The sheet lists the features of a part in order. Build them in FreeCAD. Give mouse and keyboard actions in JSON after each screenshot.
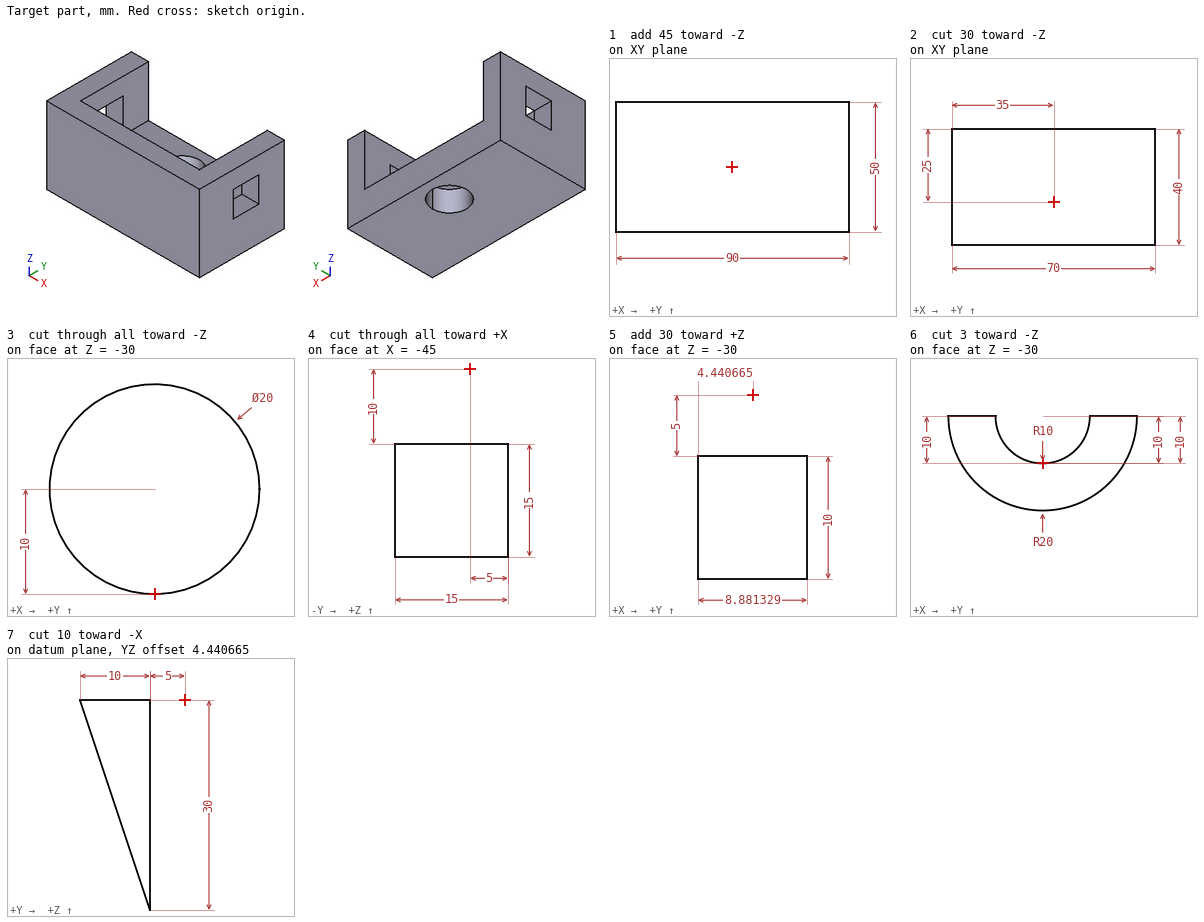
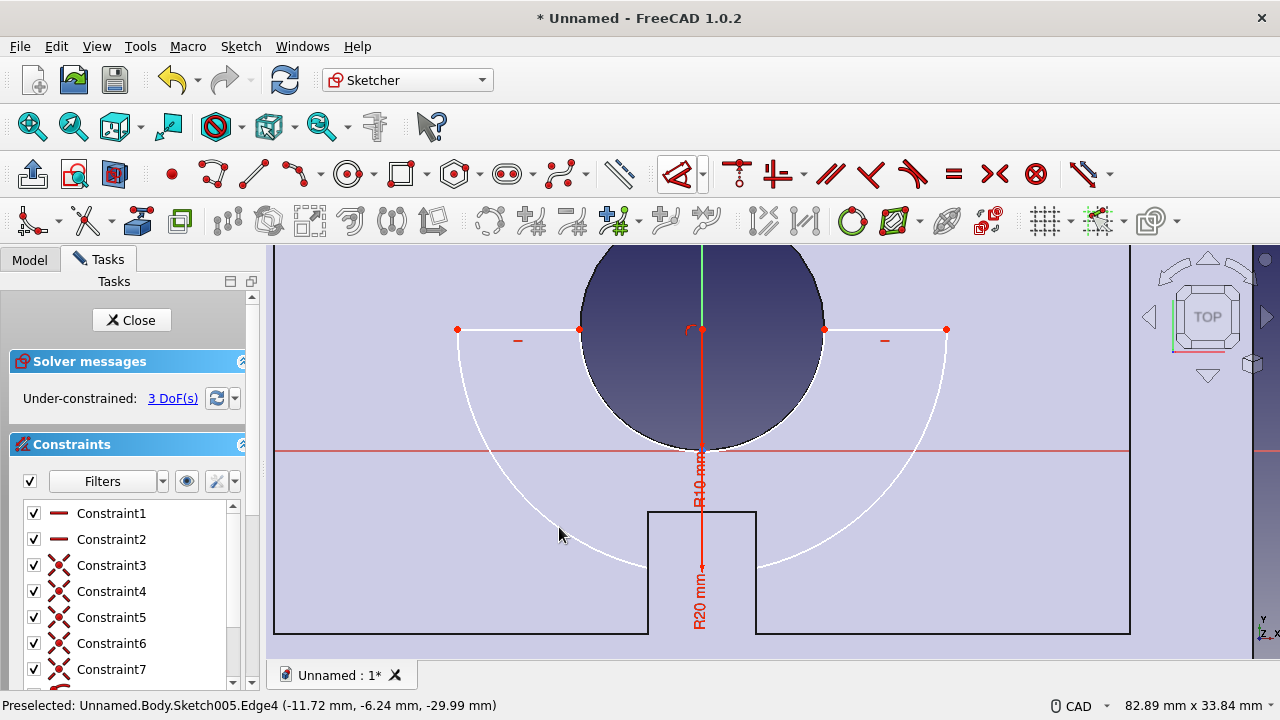
{"action": "left_click", "coordinate": [947, 330]}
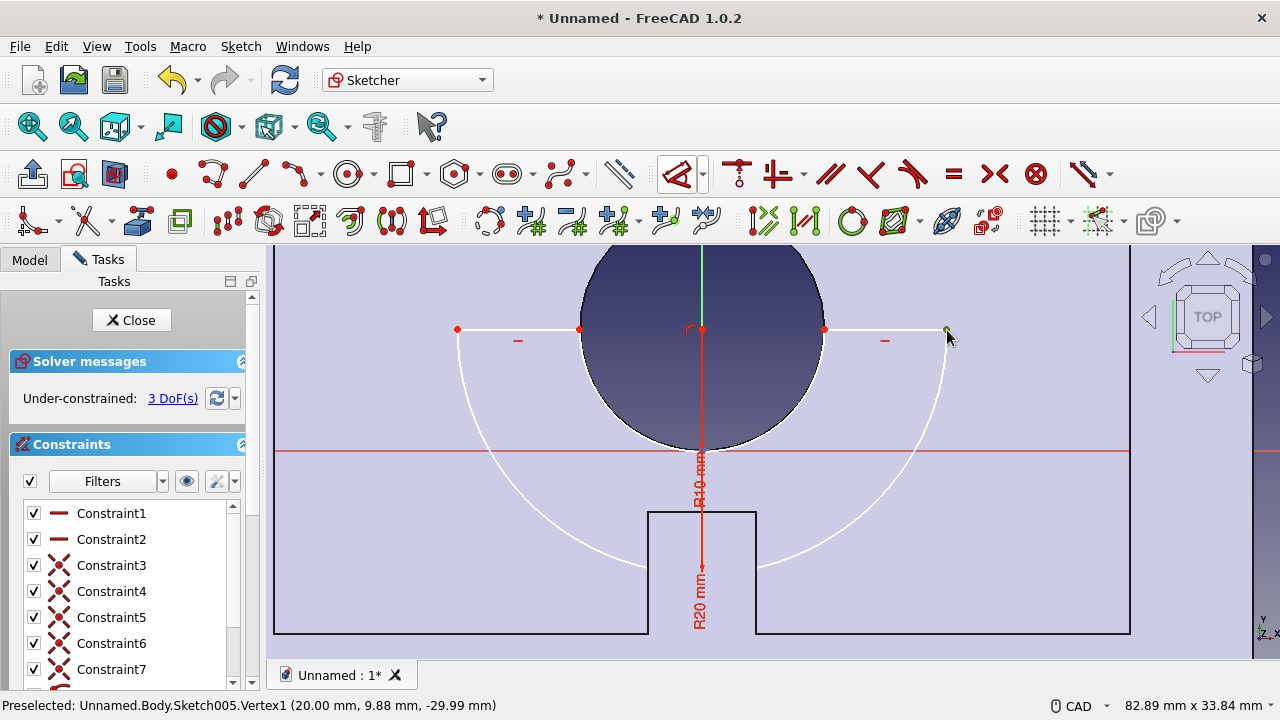
{"action": "key", "text": "i"}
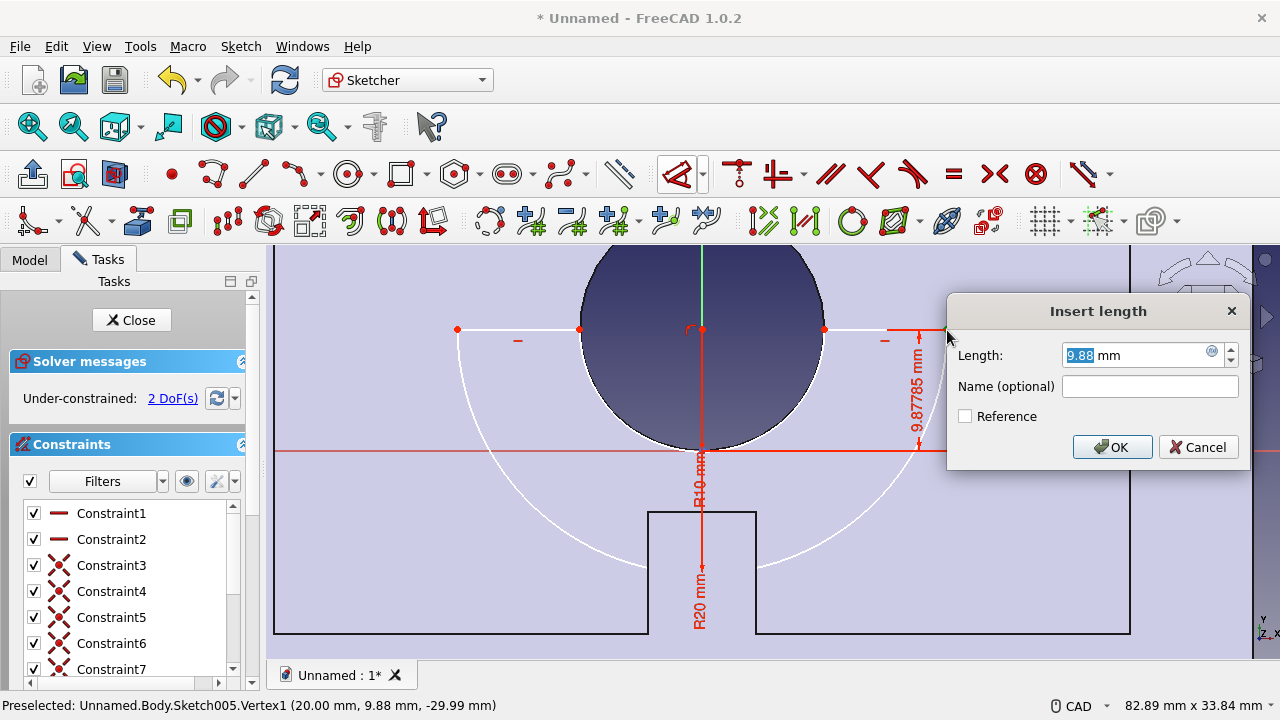
{"action": "type", "text": "10"}
{"action": "key", "text": "Return"}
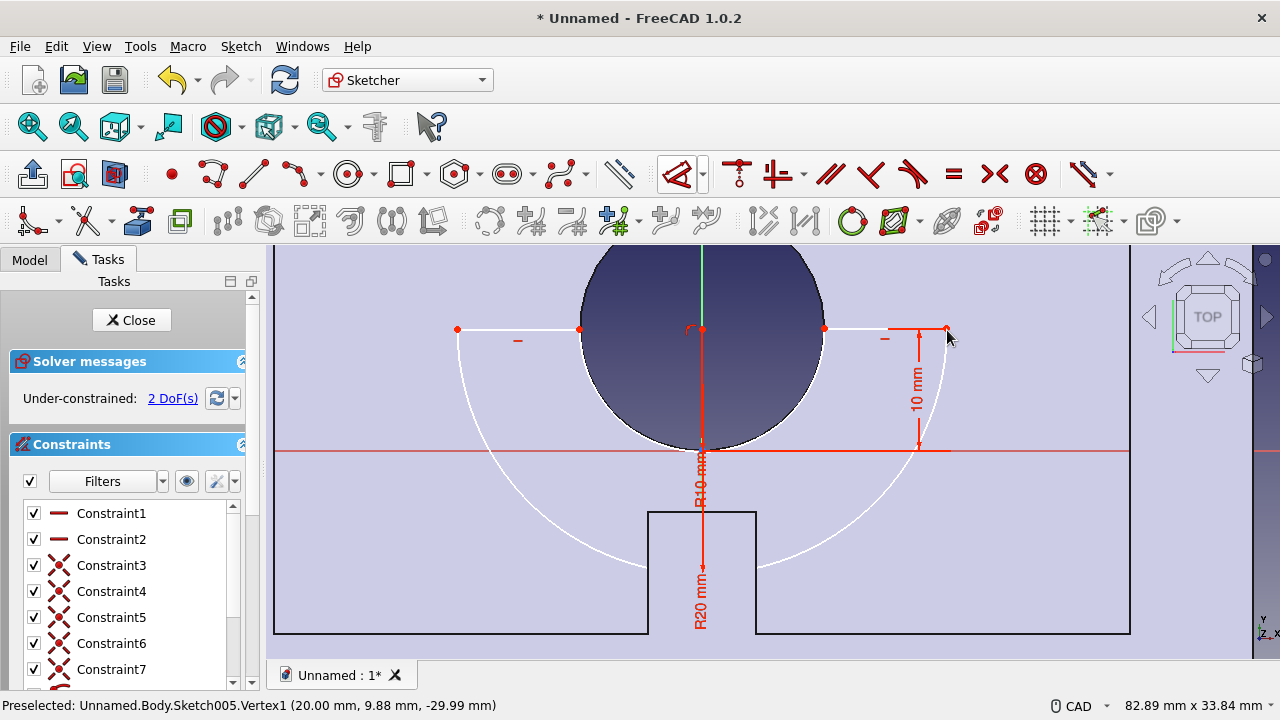
{"action": "left_click", "coordinate": [580, 330]}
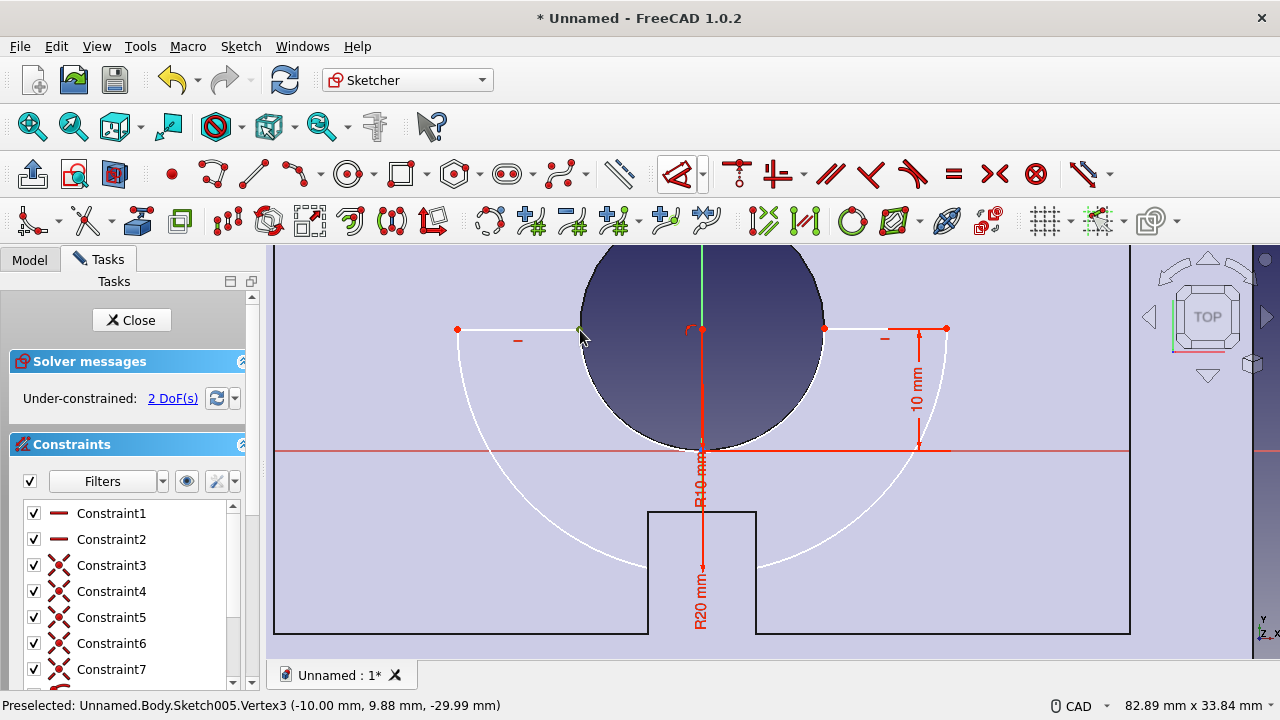
{"action": "key", "text": "i"}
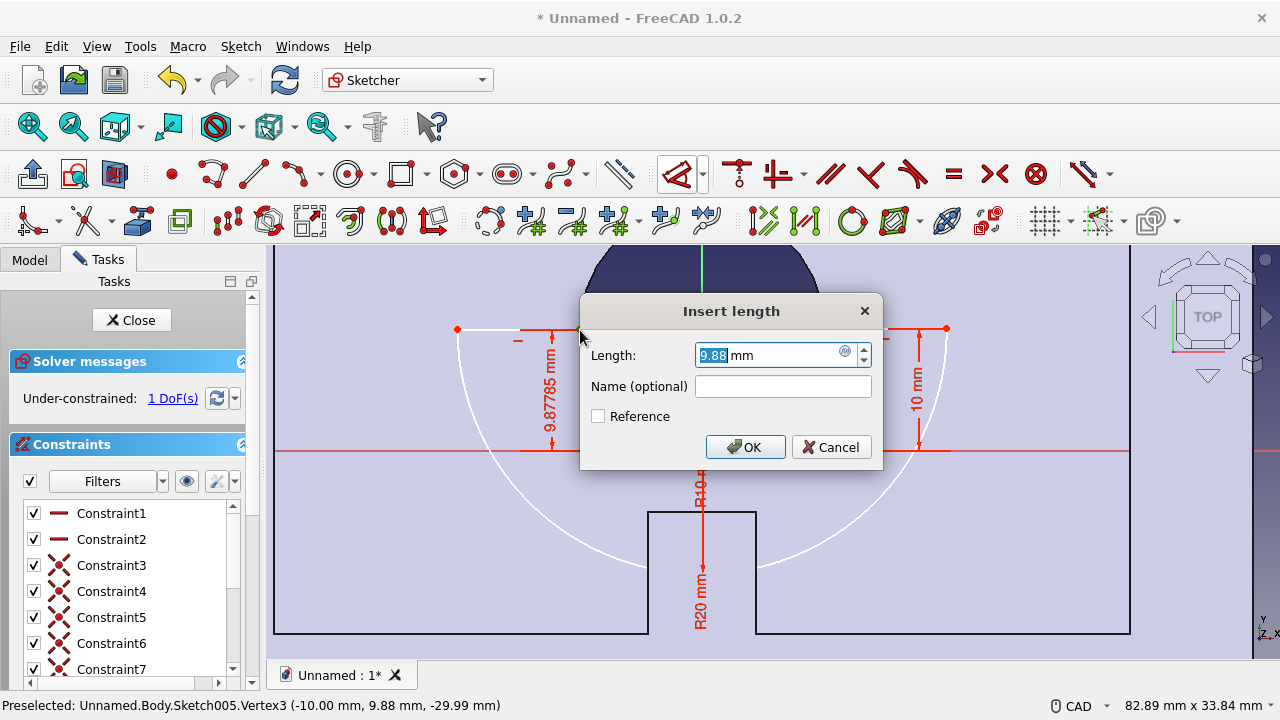
{"action": "type", "text": "10"}
{"action": "key", "text": "Return"}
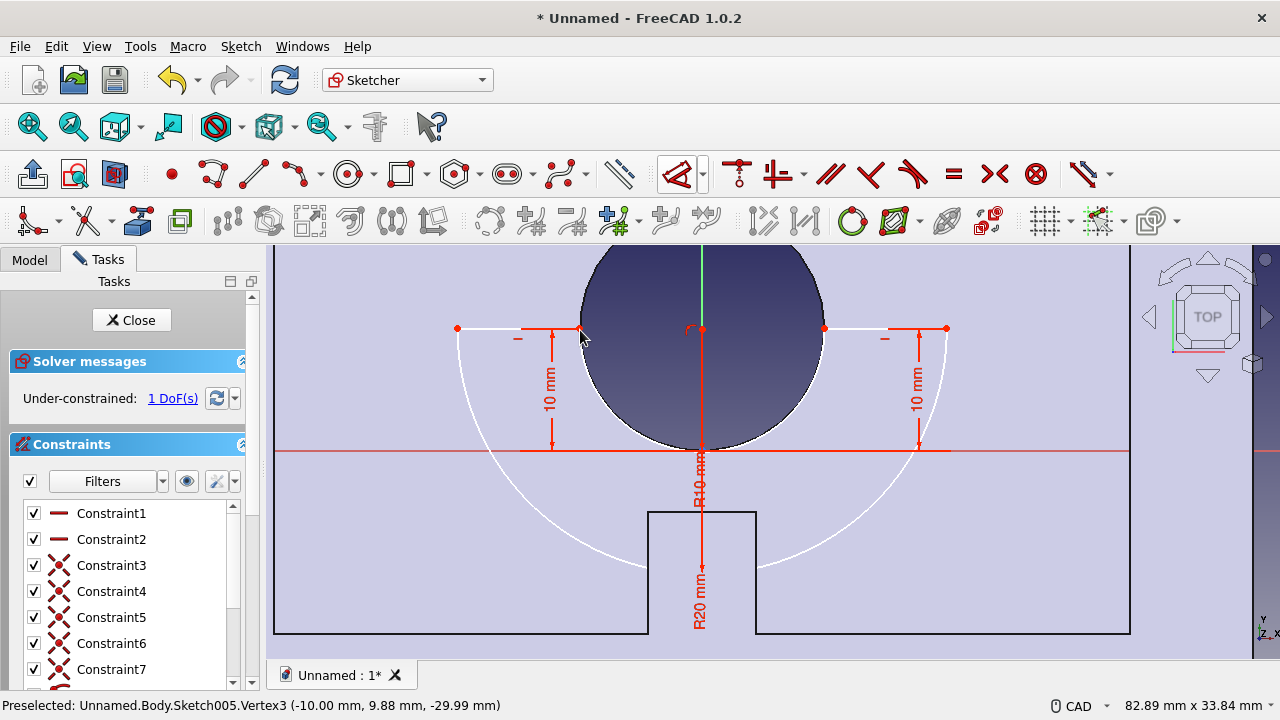
{"action": "left_click", "coordinate": [702, 329]}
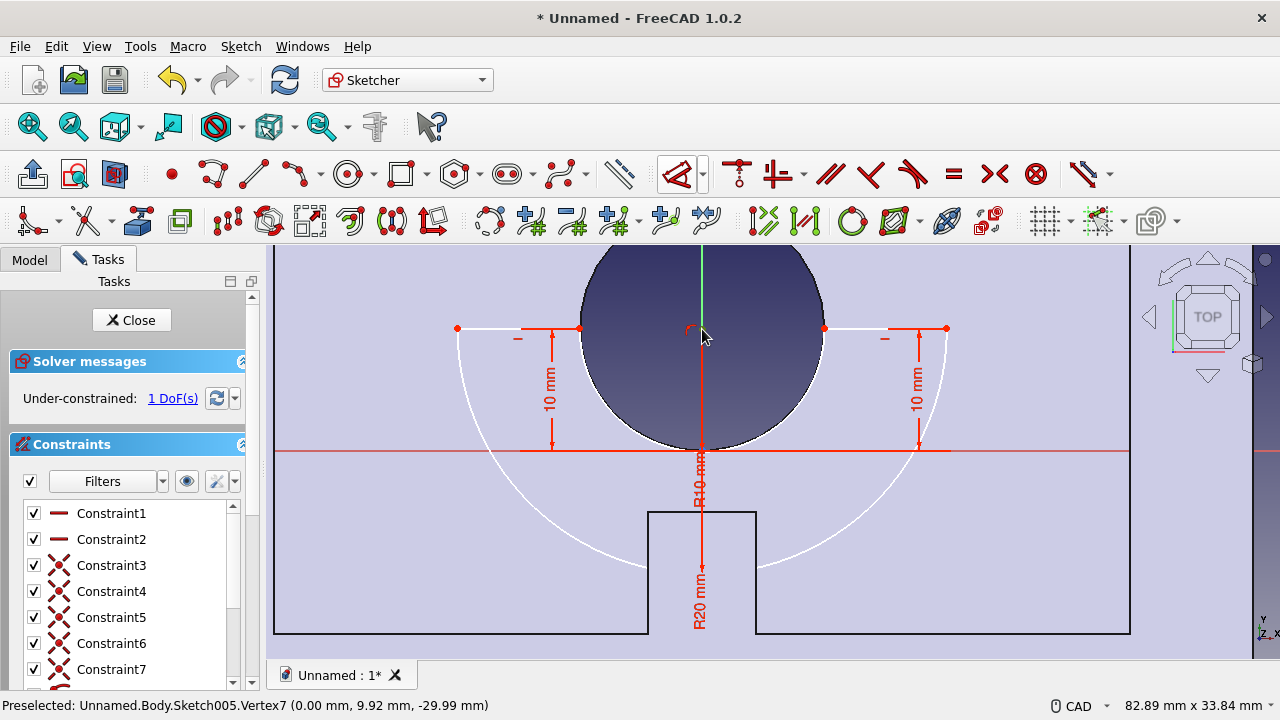
{"action": "key", "text": "i"}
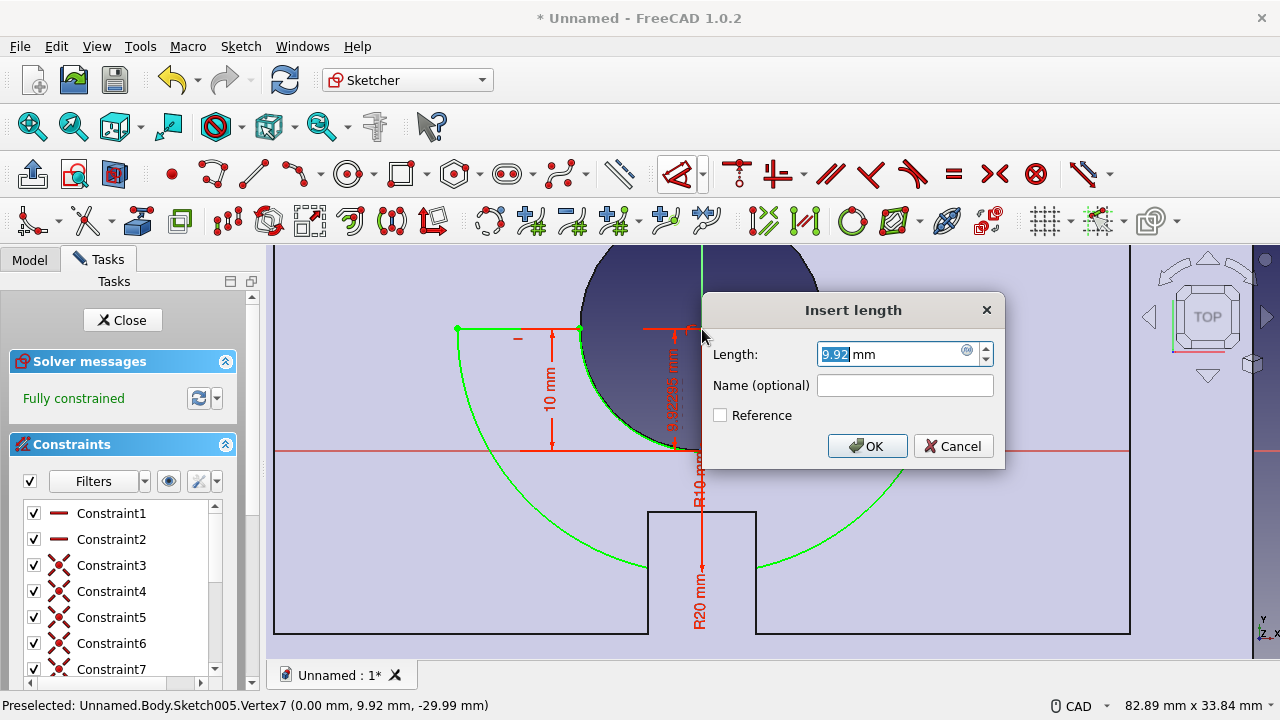
{"action": "type", "text": "10"}
{"action": "key", "text": "Return"}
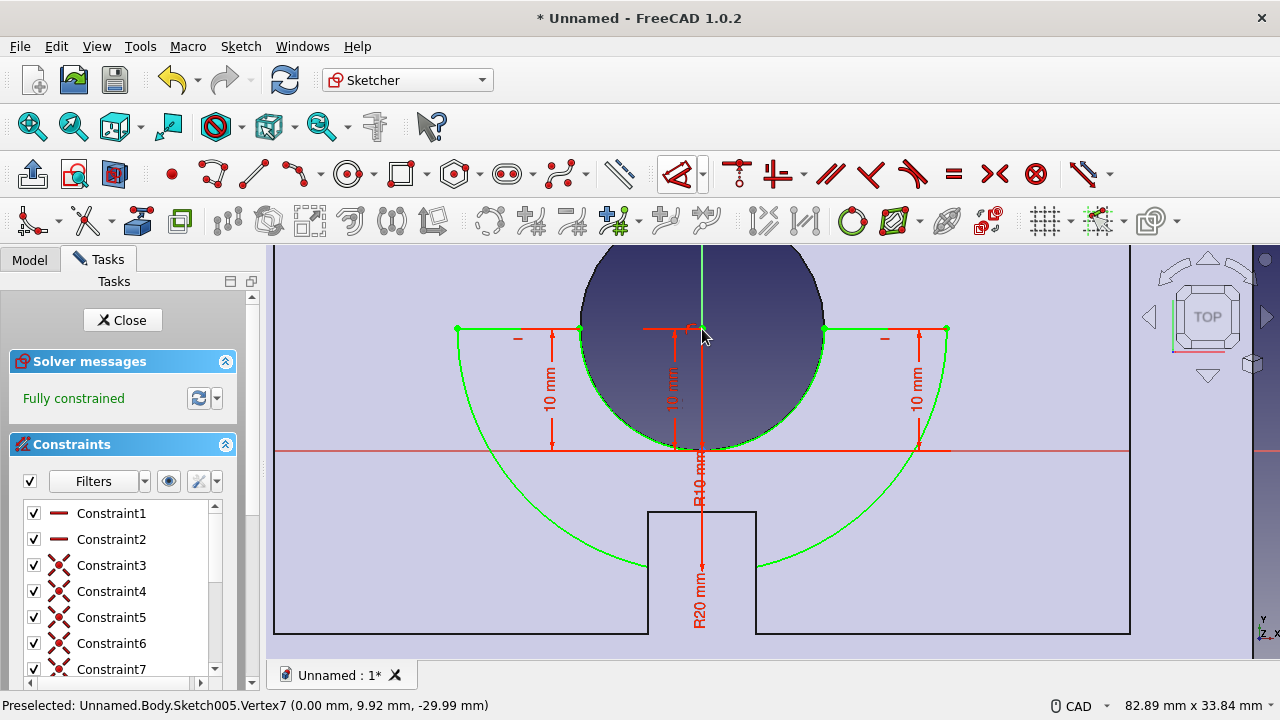
{"action": "left_click", "coordinate": [123, 320]}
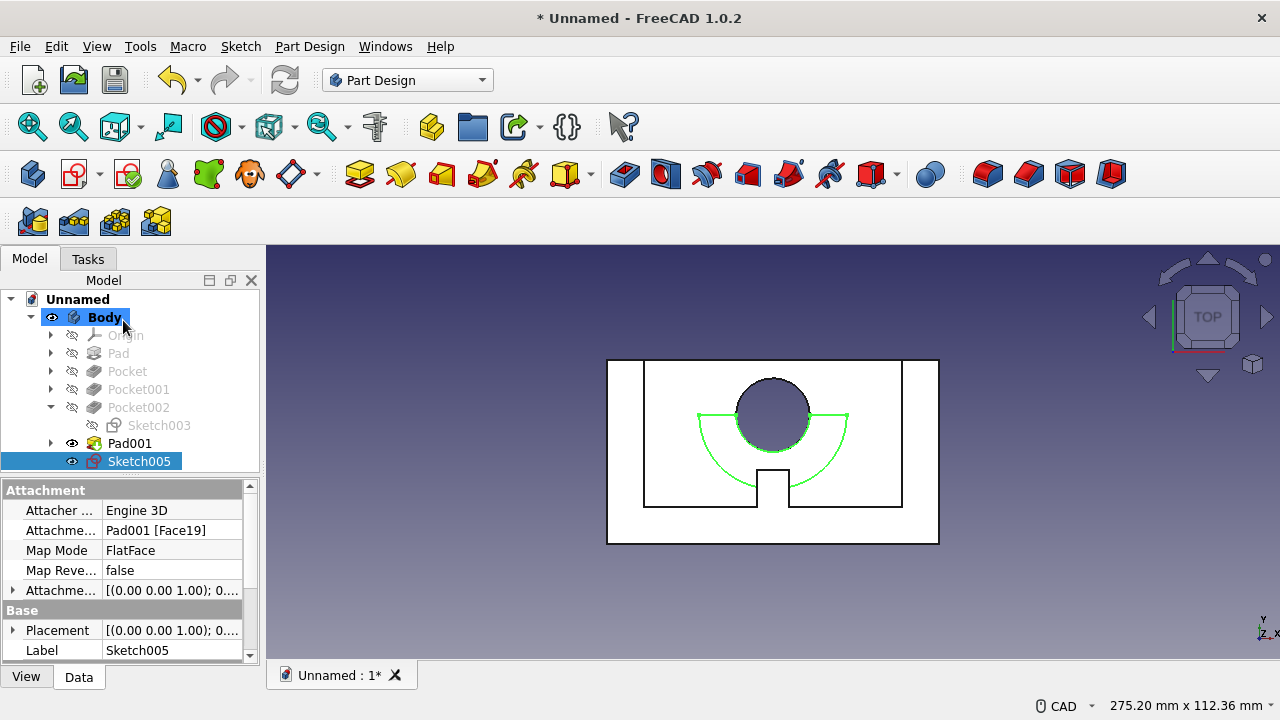
{"action": "left_click", "coordinate": [625, 174]}